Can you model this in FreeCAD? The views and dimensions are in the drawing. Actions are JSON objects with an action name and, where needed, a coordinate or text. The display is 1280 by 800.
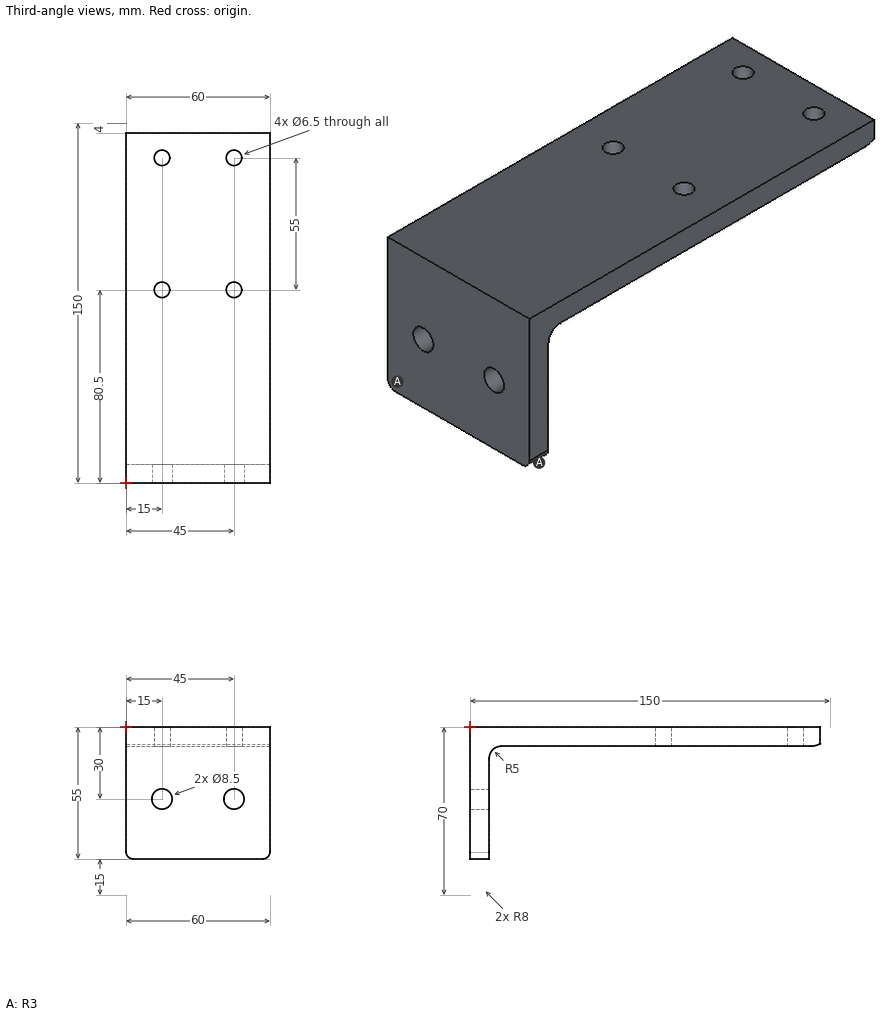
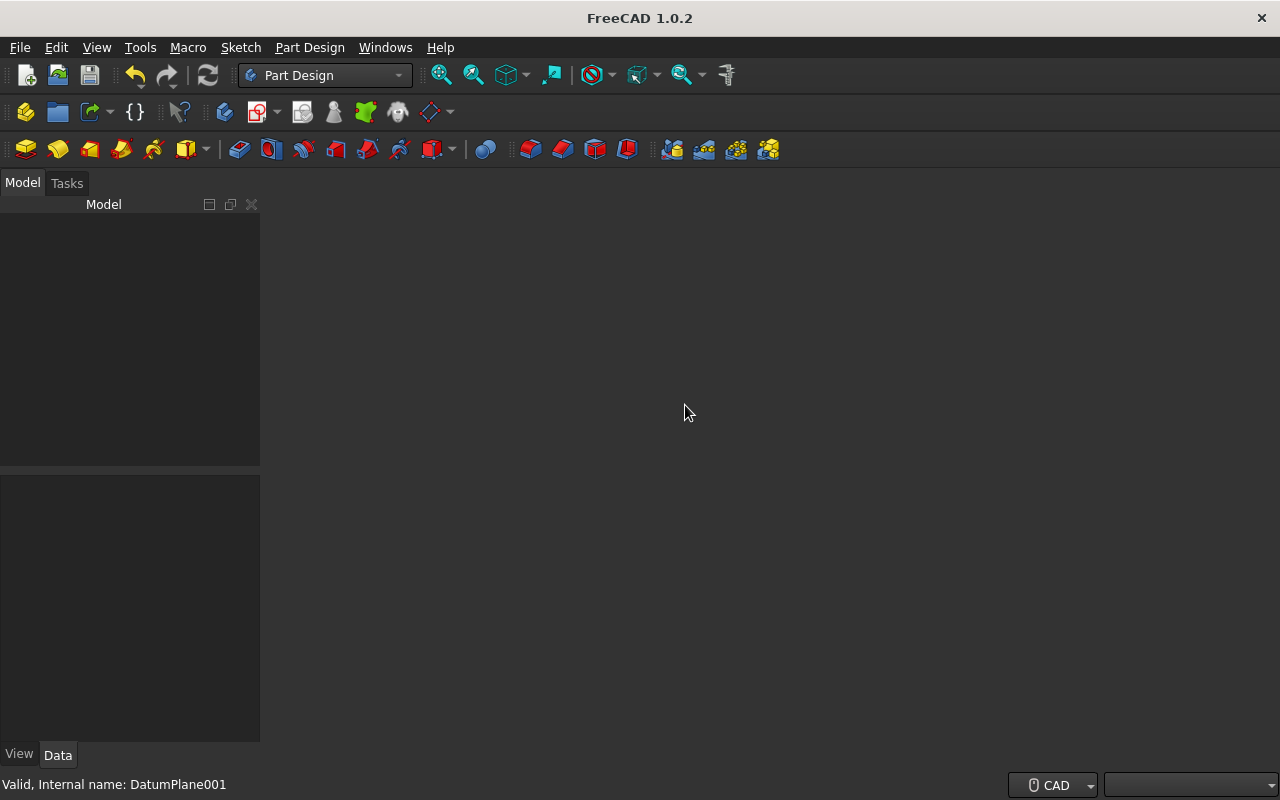
{"action": "left_click", "coordinate": [26, 76]}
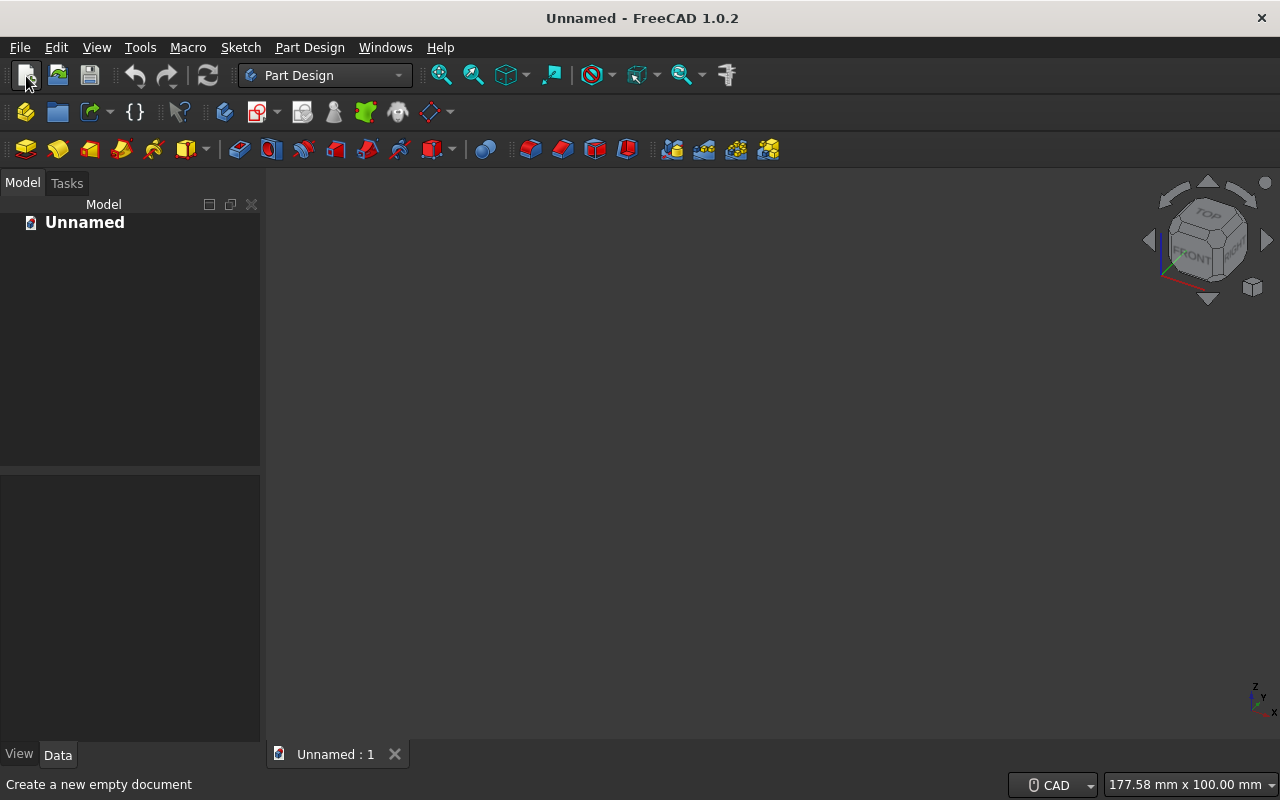
{"action": "left_click", "coordinate": [258, 112]}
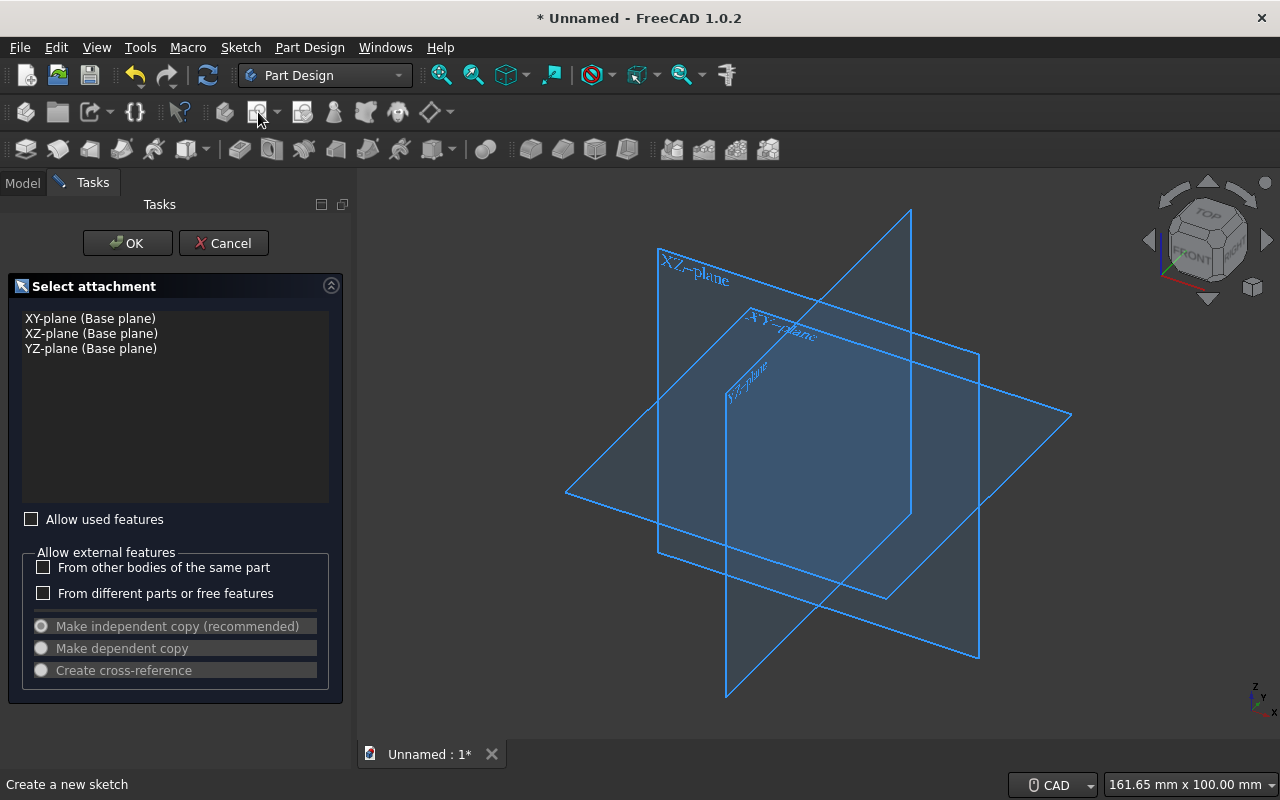
{"action": "left_click", "coordinate": [82, 348]}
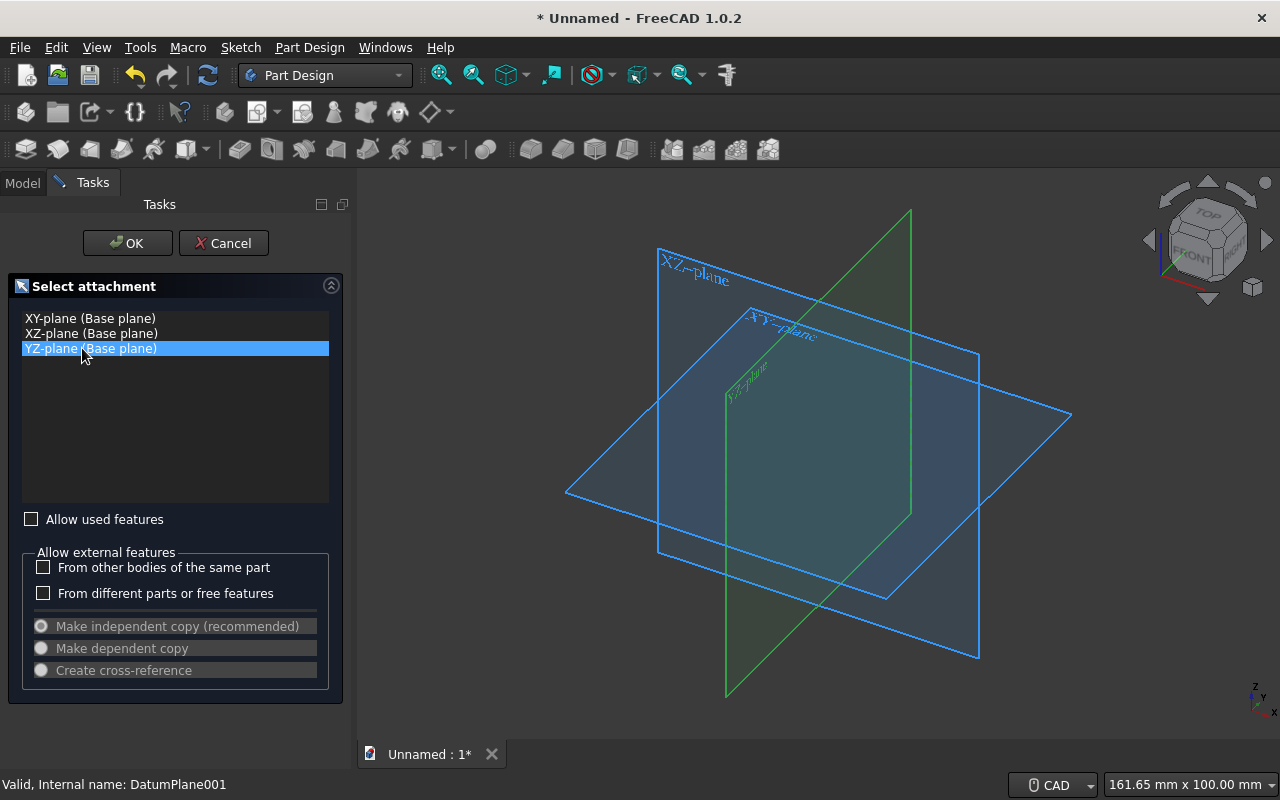
{"action": "left_click", "coordinate": [128, 243]}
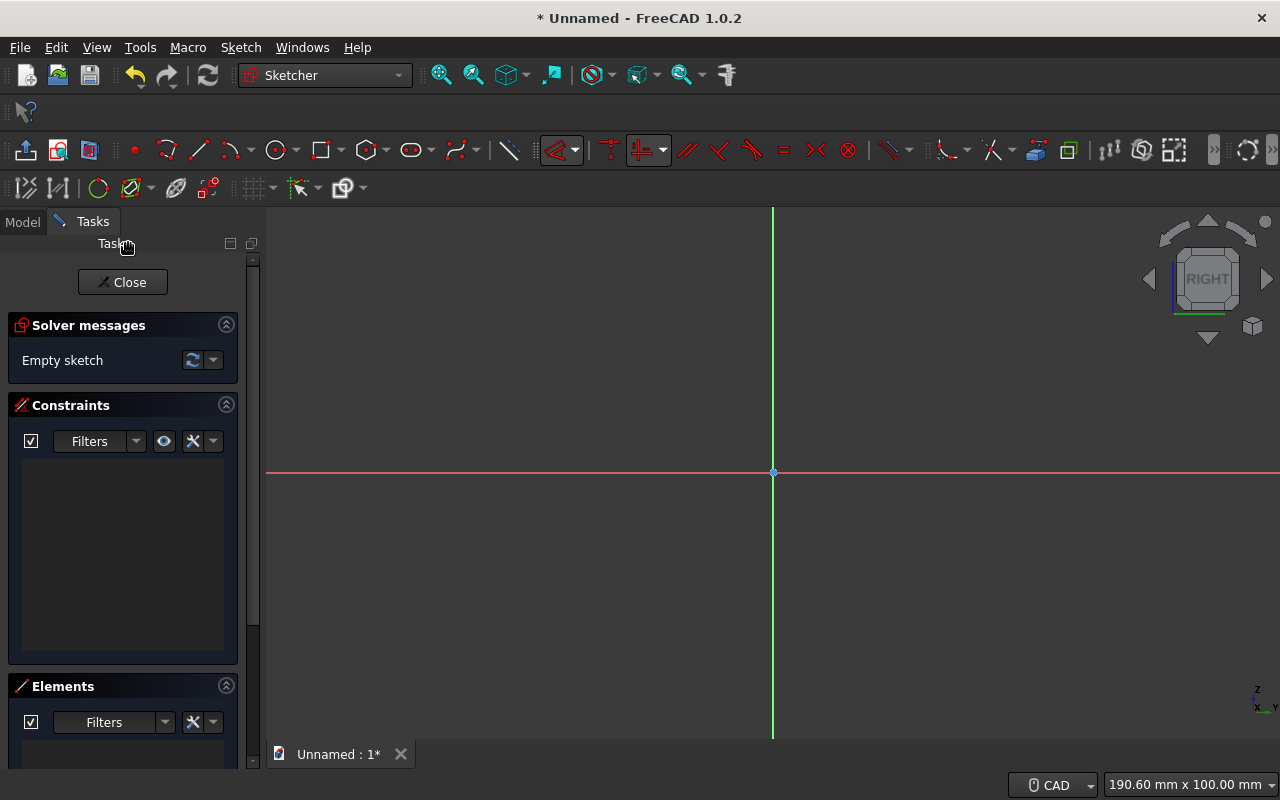
{"action": "scroll", "coordinate": [294, 247], "scroll_direction": "down", "scroll_amount": 3}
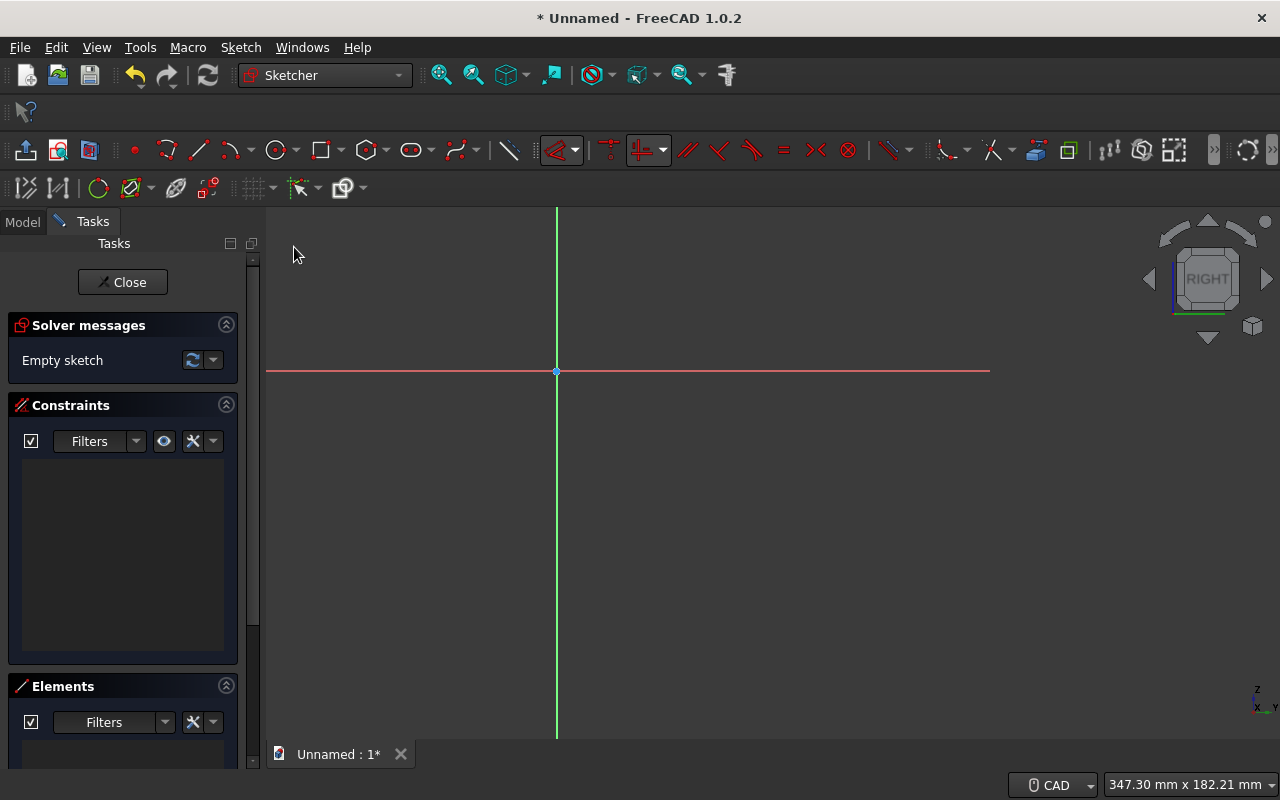
{"action": "key", "text": "g m"}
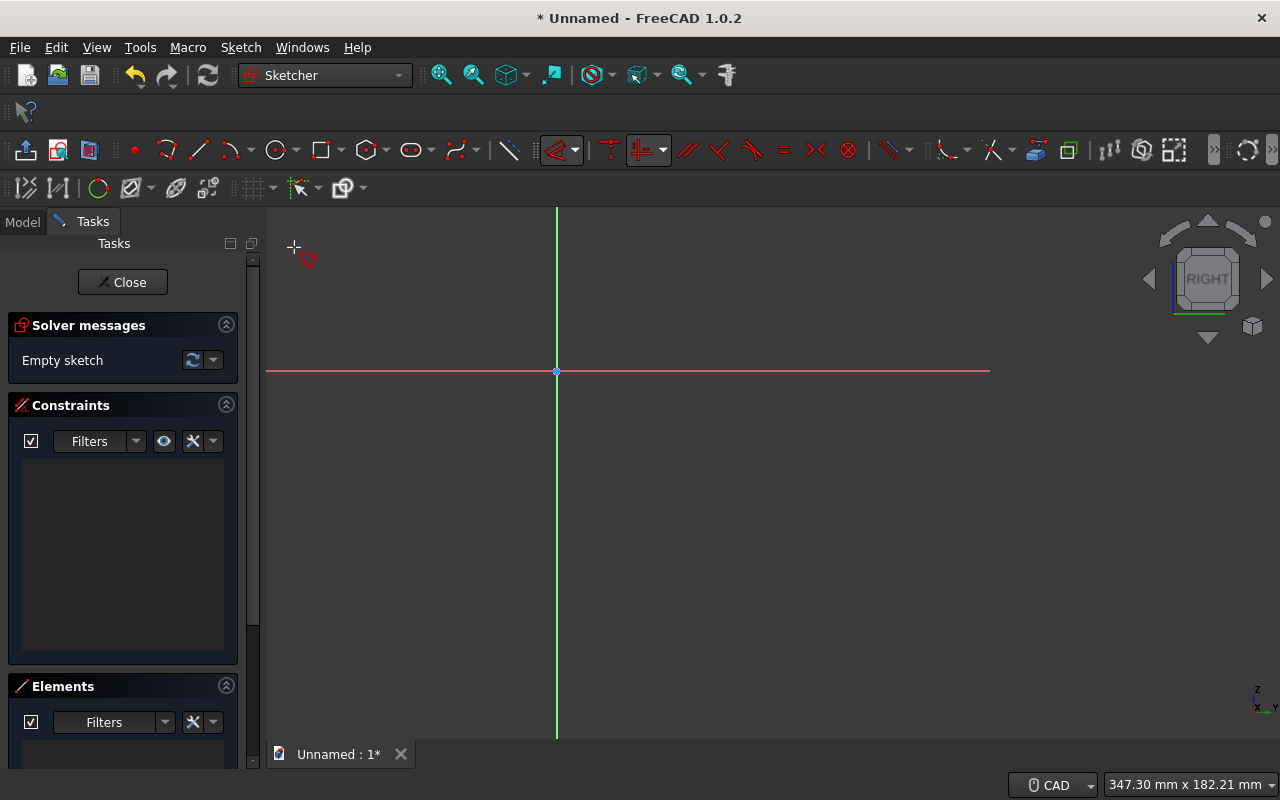
{"action": "left_click", "coordinate": [995, 371]}
{"action": "left_click", "coordinate": [557, 371]}
{"action": "left_click", "coordinate": [566, 575]}
{"action": "right_click", "coordinate": [566, 575]}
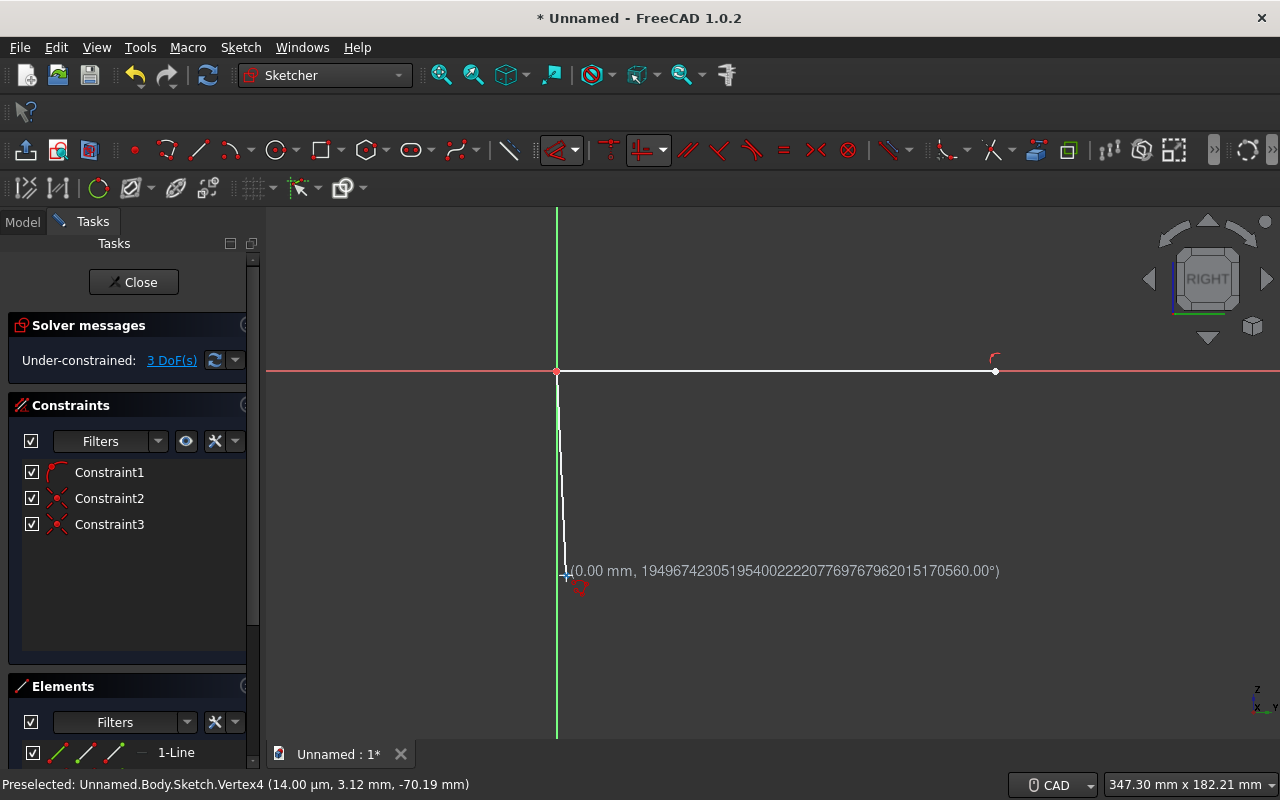
{"action": "key", "text": "g l"}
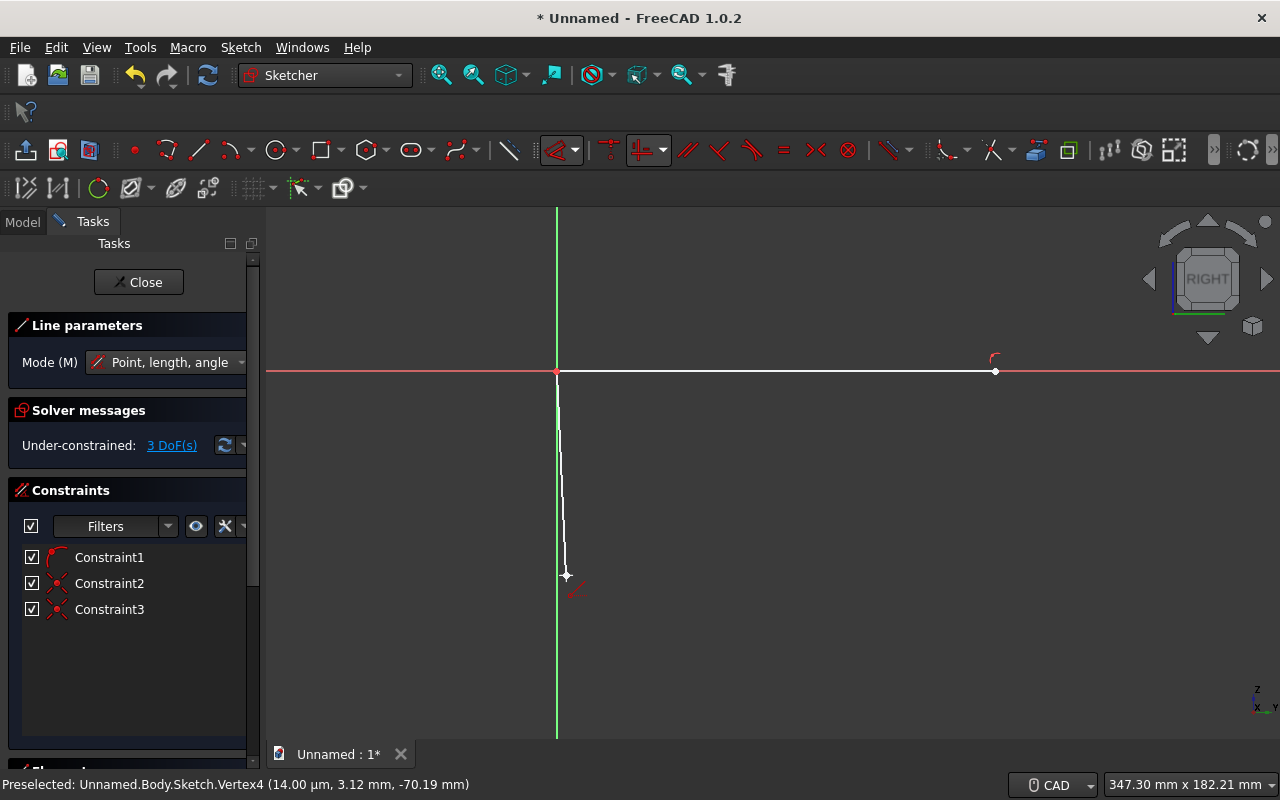
{"action": "left_click", "coordinate": [580, 552]}
{"action": "left_click", "coordinate": [580, 409]}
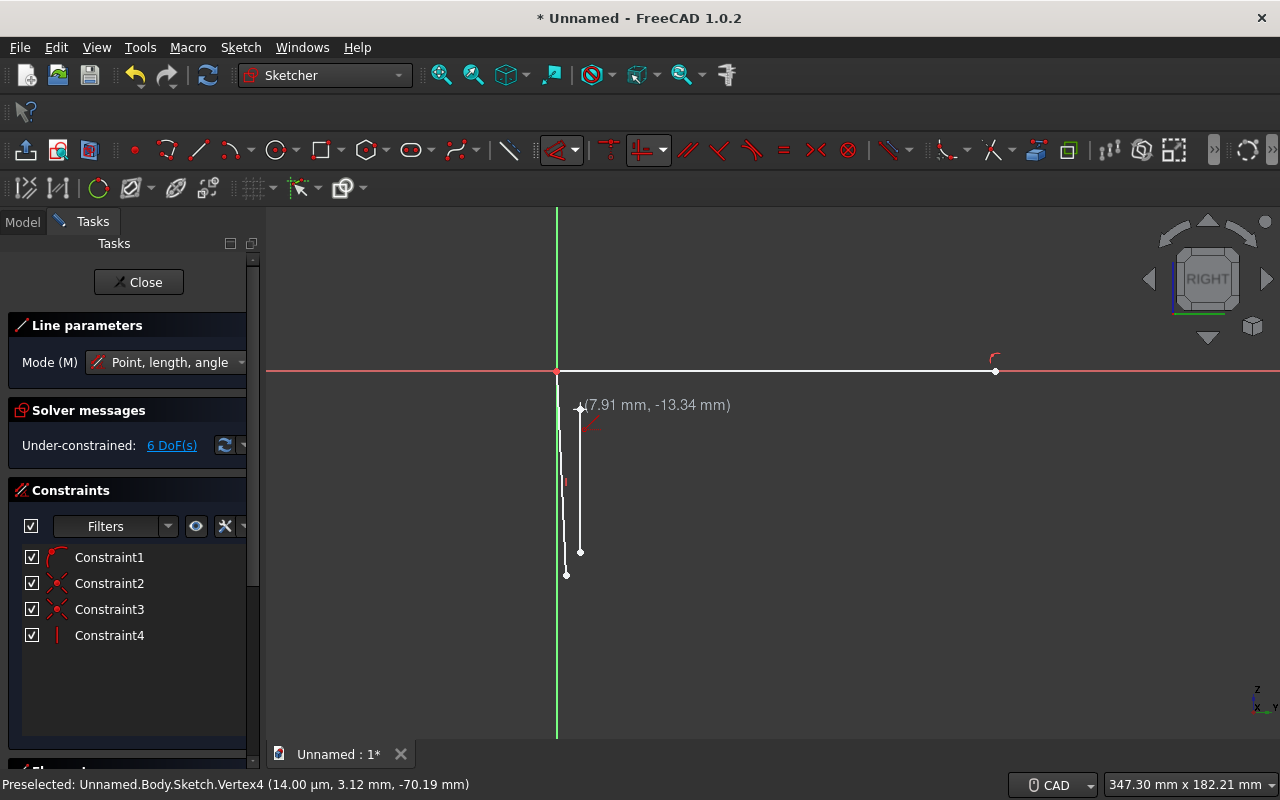
{"action": "left_click", "coordinate": [595, 394]}
{"action": "left_click", "coordinate": [971, 394]}